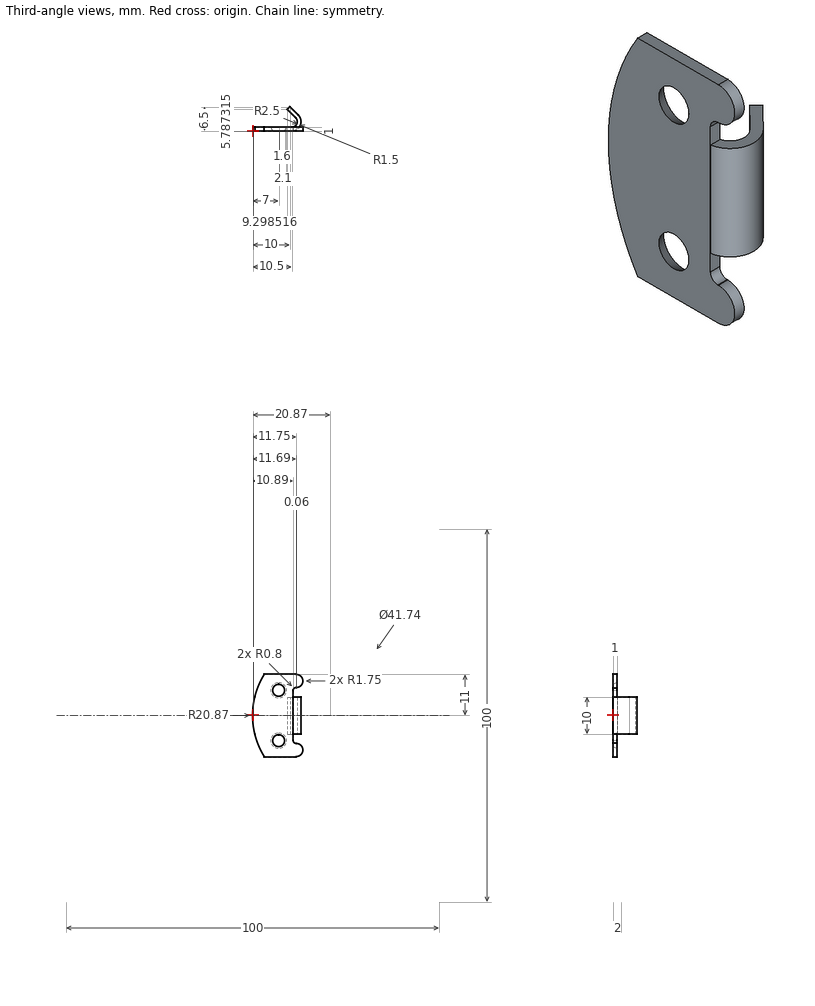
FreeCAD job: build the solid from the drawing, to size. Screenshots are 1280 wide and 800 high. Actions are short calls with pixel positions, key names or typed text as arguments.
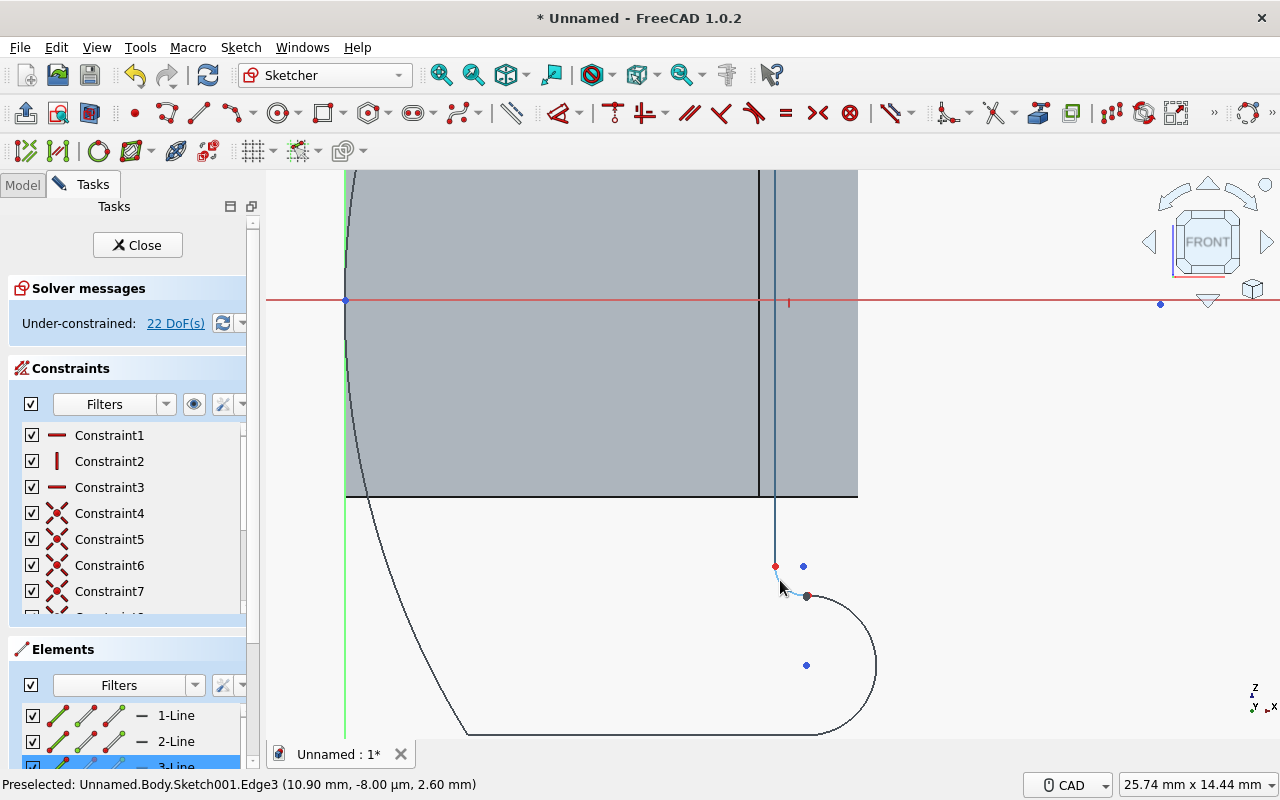
click(778, 580)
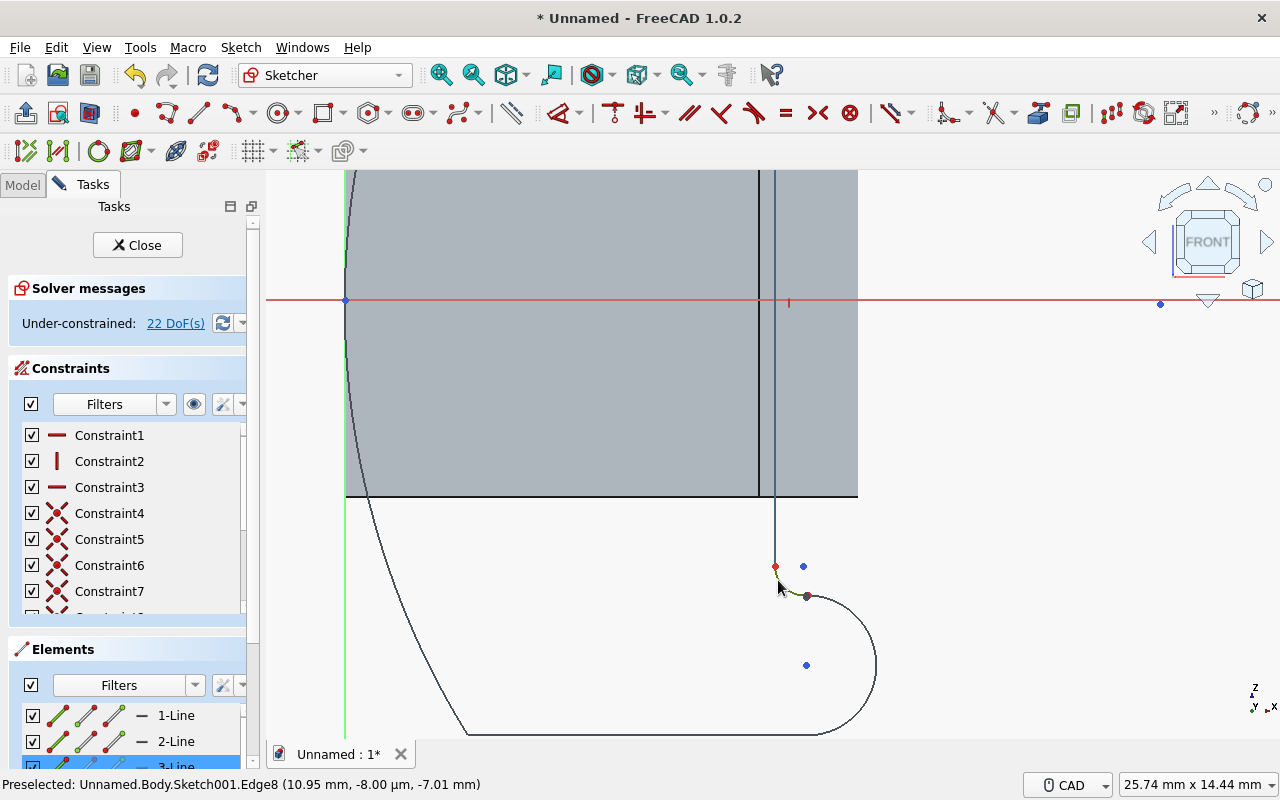
key(t)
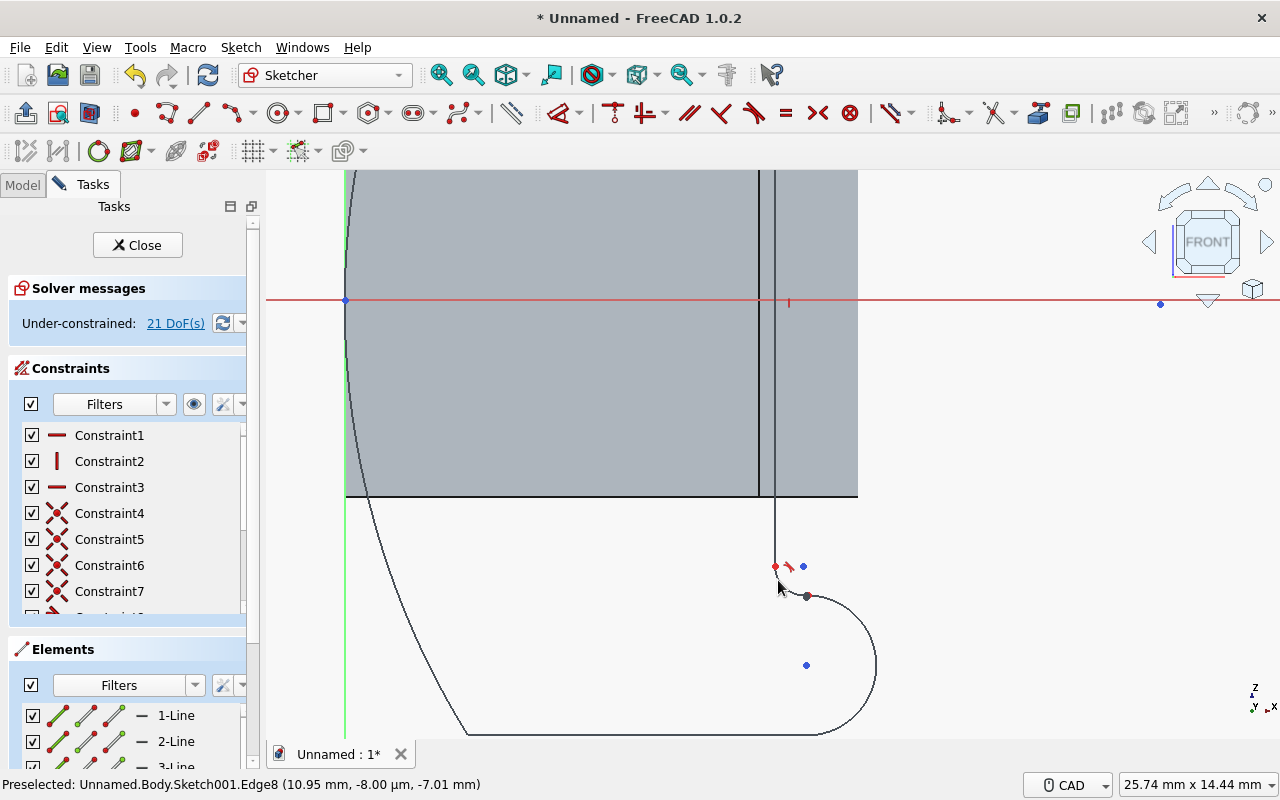
scroll(807, 596, up, 10)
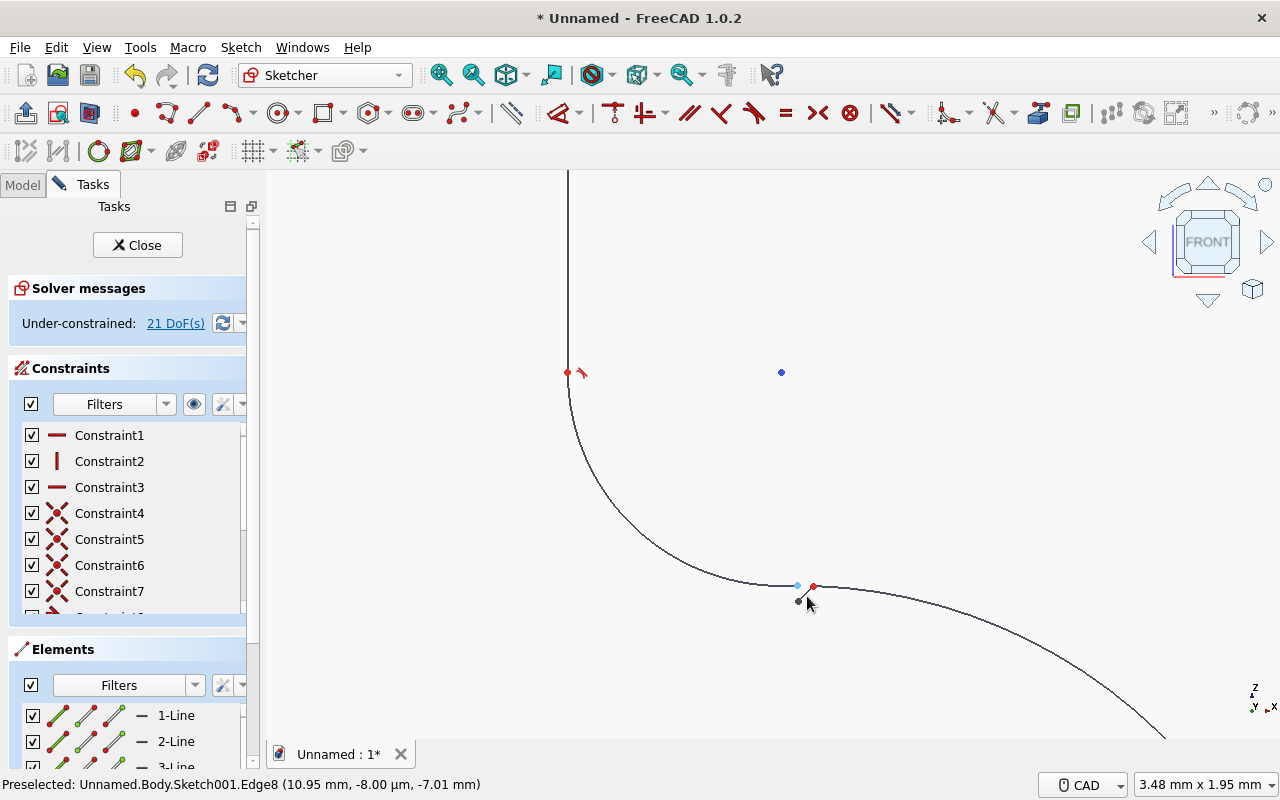
click(806, 594)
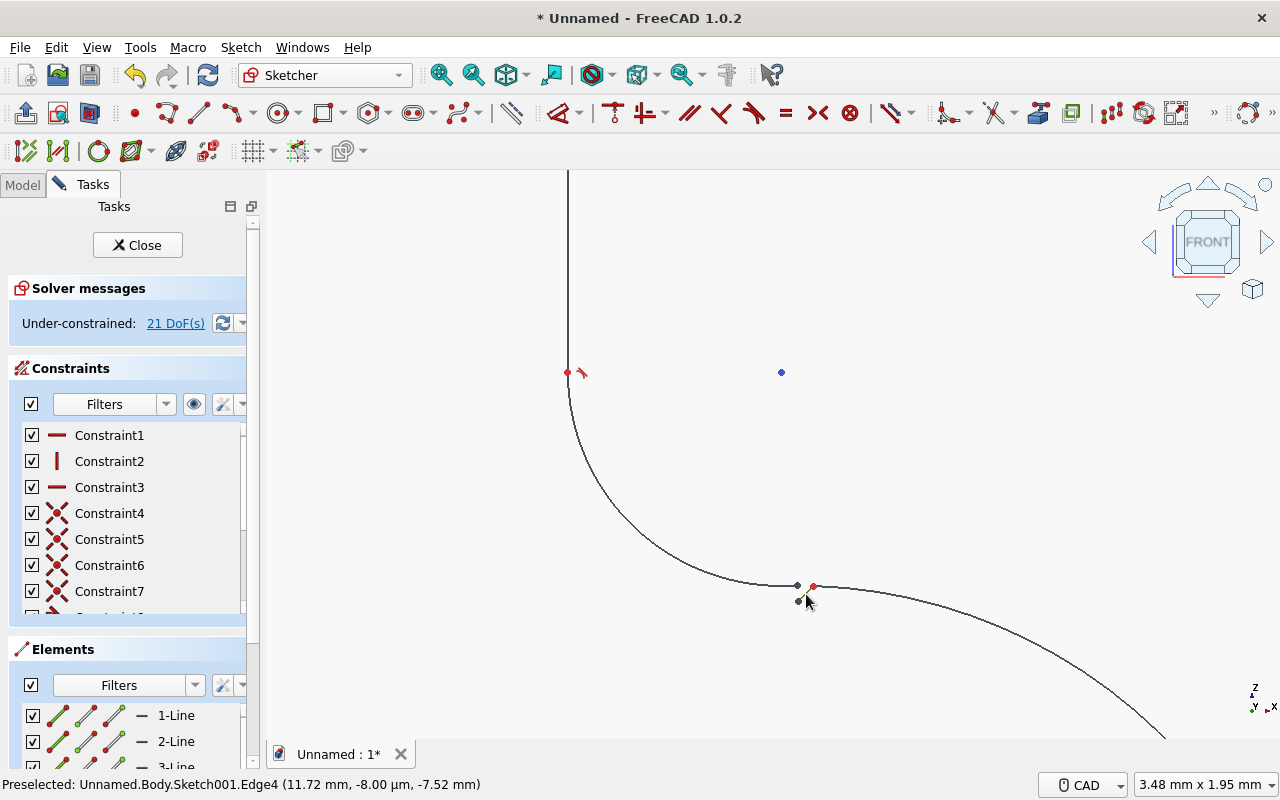
scroll(792, 587, down, 14)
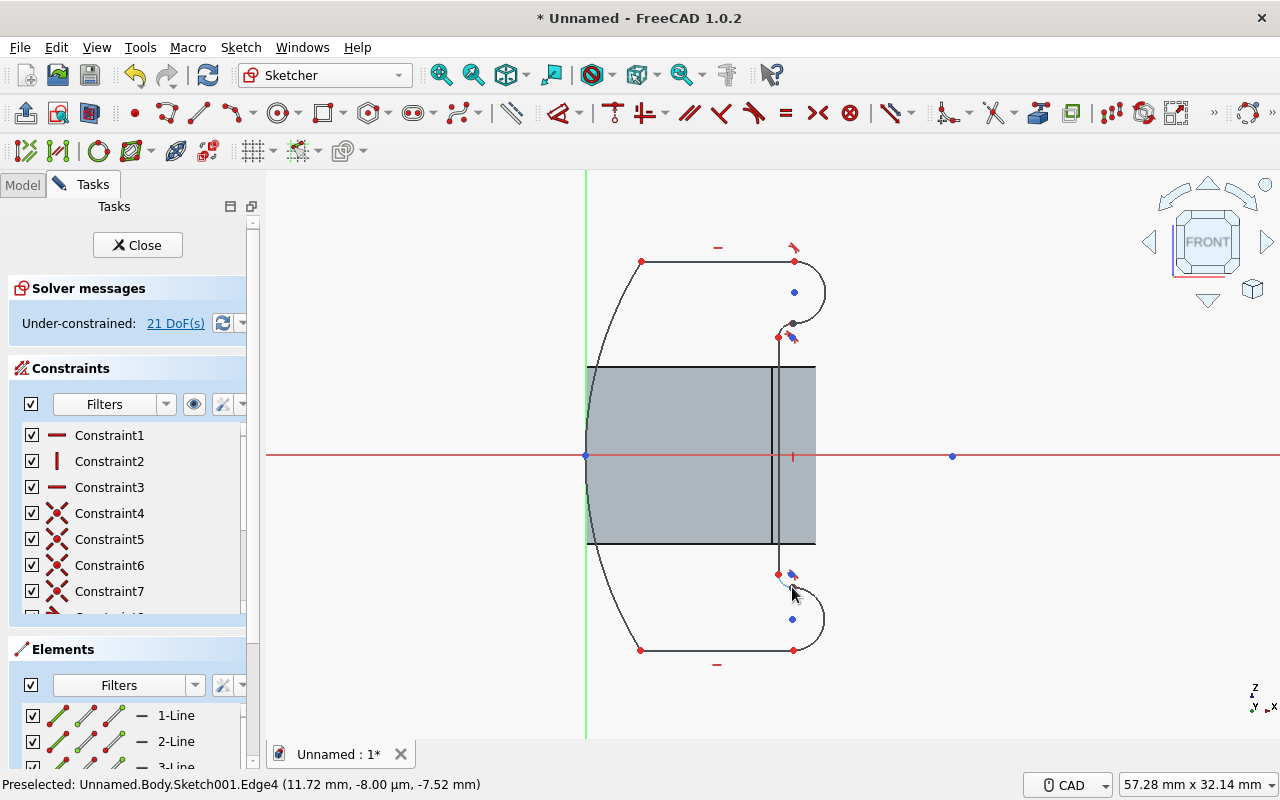
scroll(780, 581, up, 4)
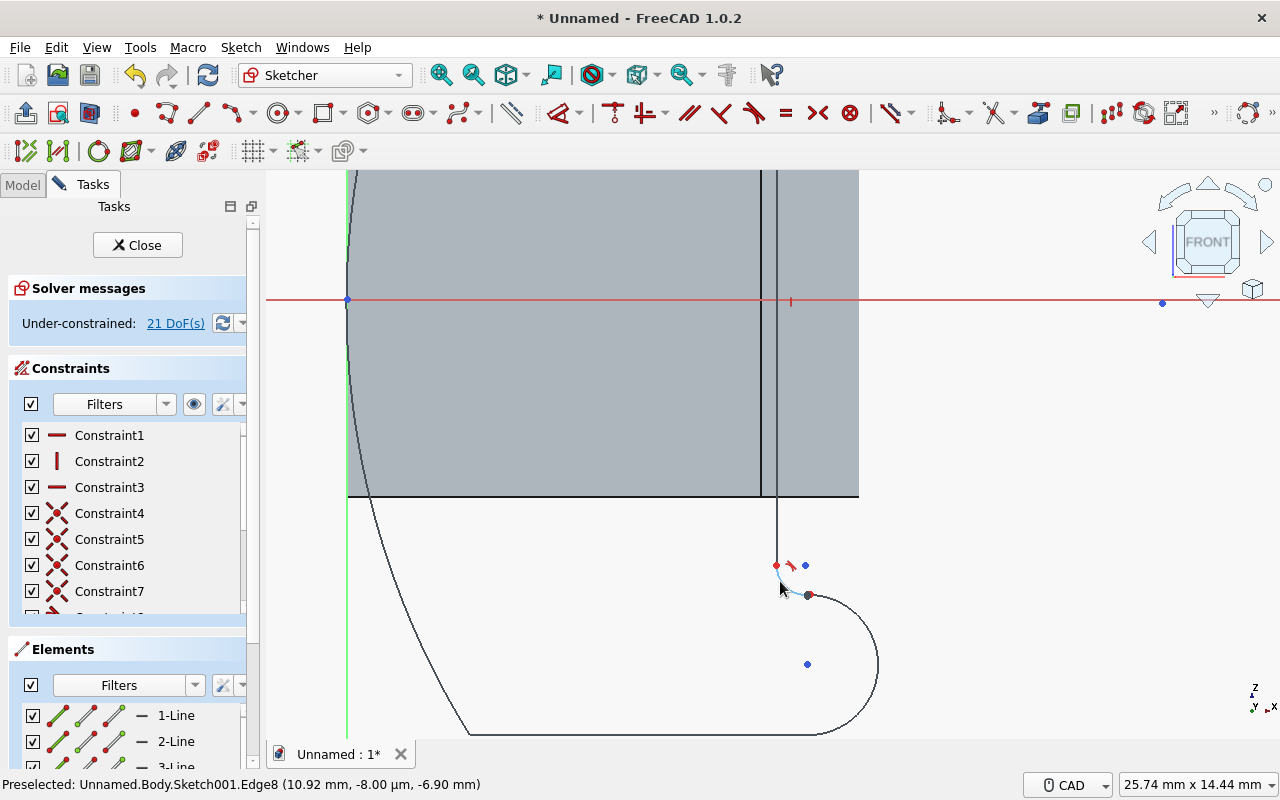
click(780, 580)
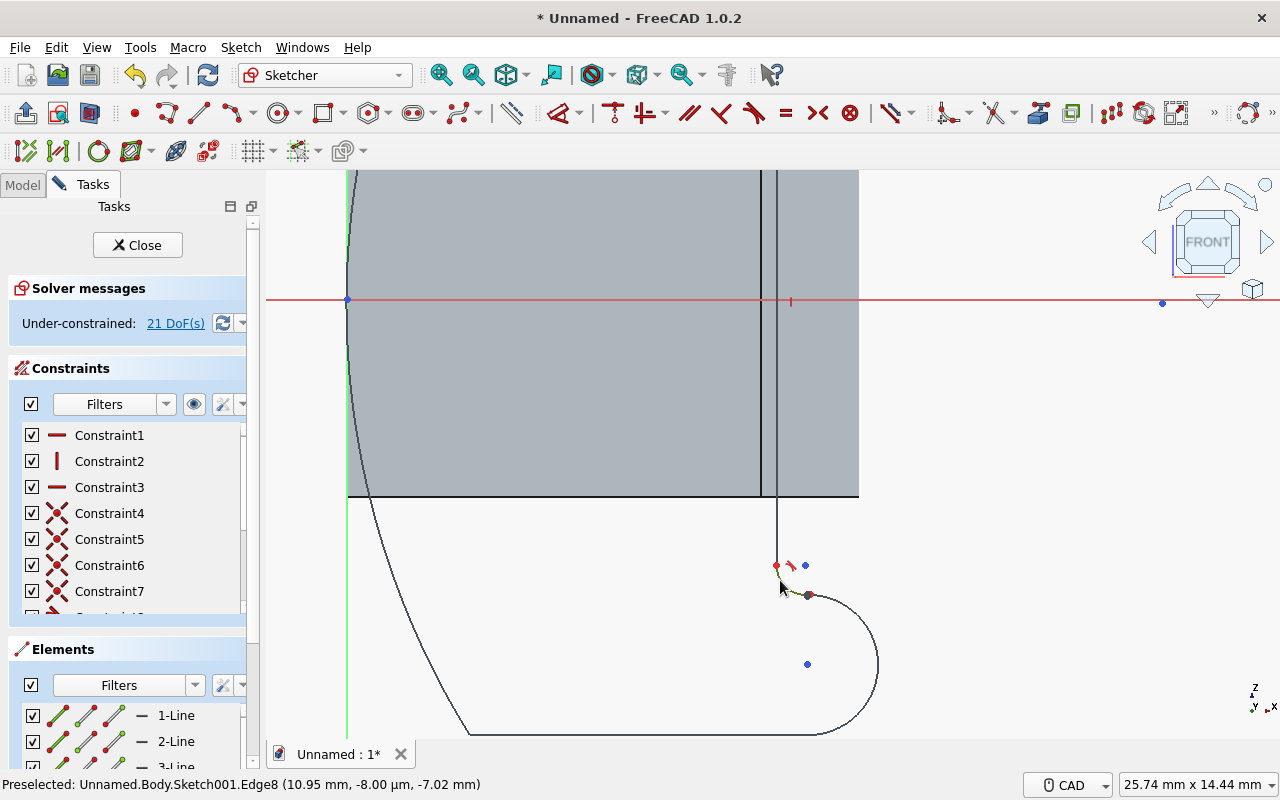
click(754, 114)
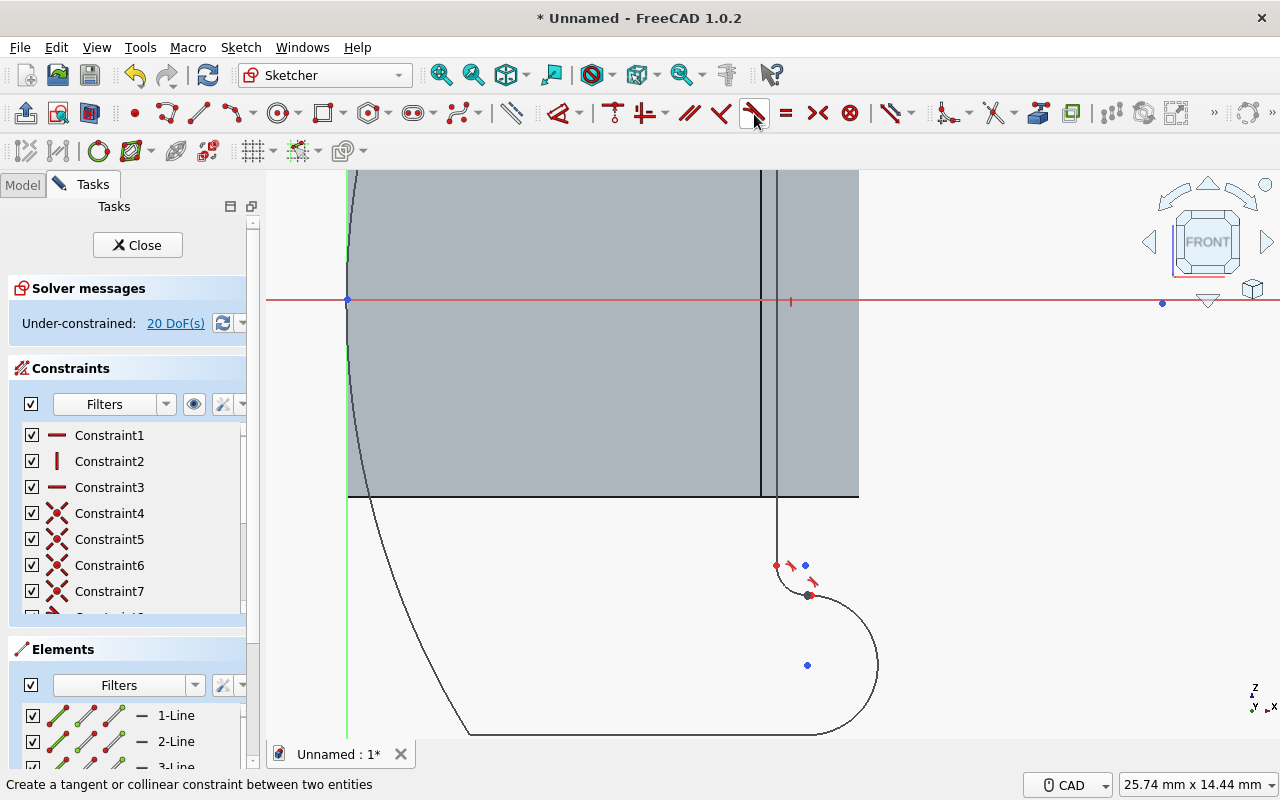
scroll(810, 596, up, 10)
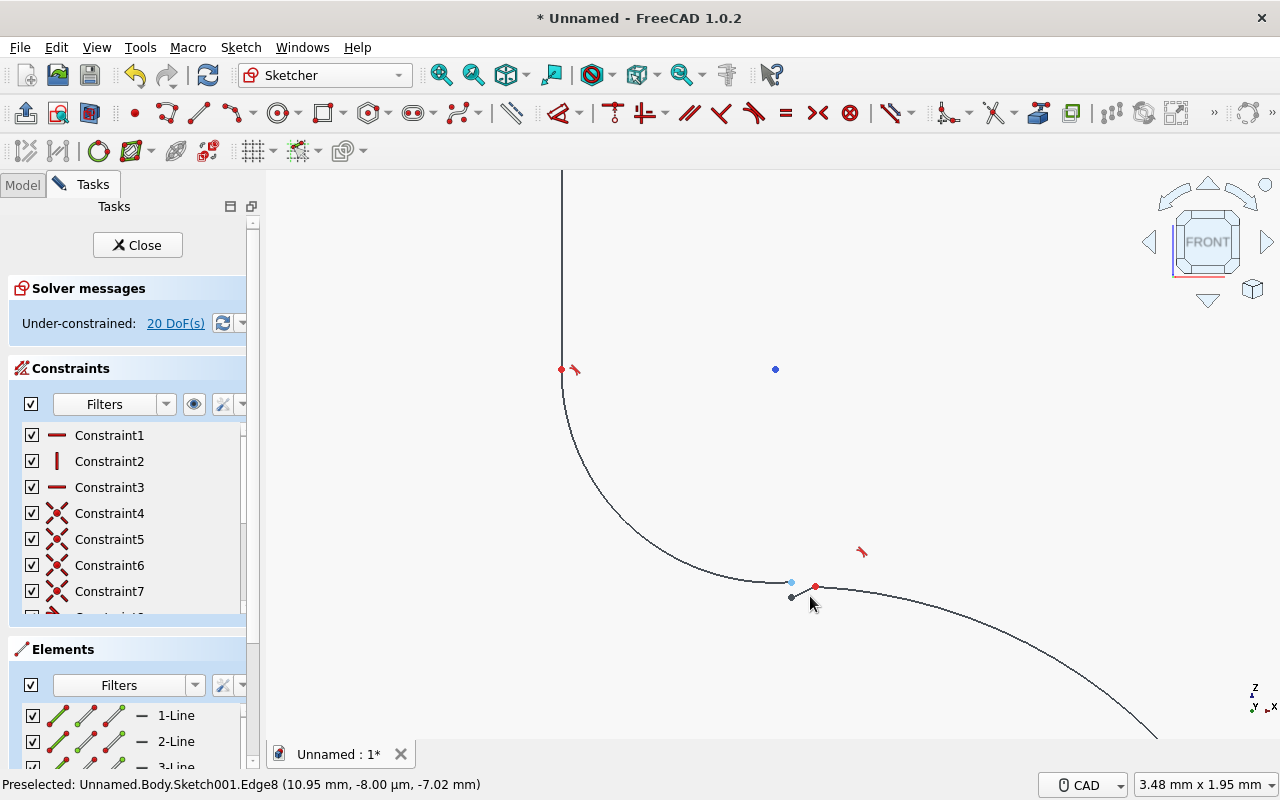
click(803, 592)